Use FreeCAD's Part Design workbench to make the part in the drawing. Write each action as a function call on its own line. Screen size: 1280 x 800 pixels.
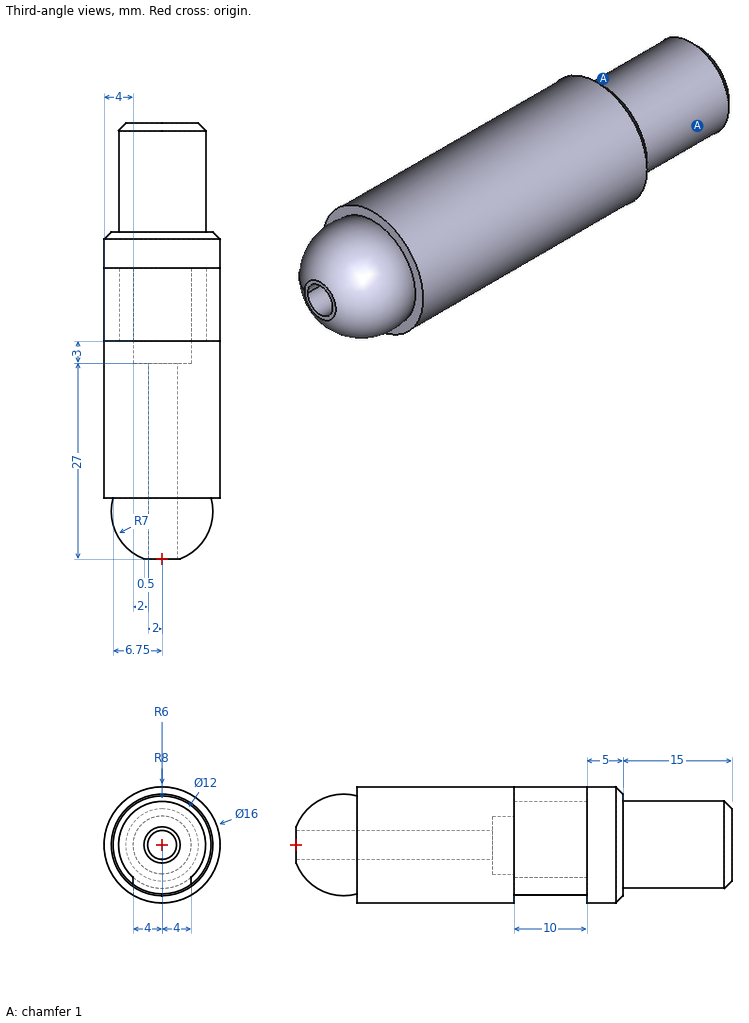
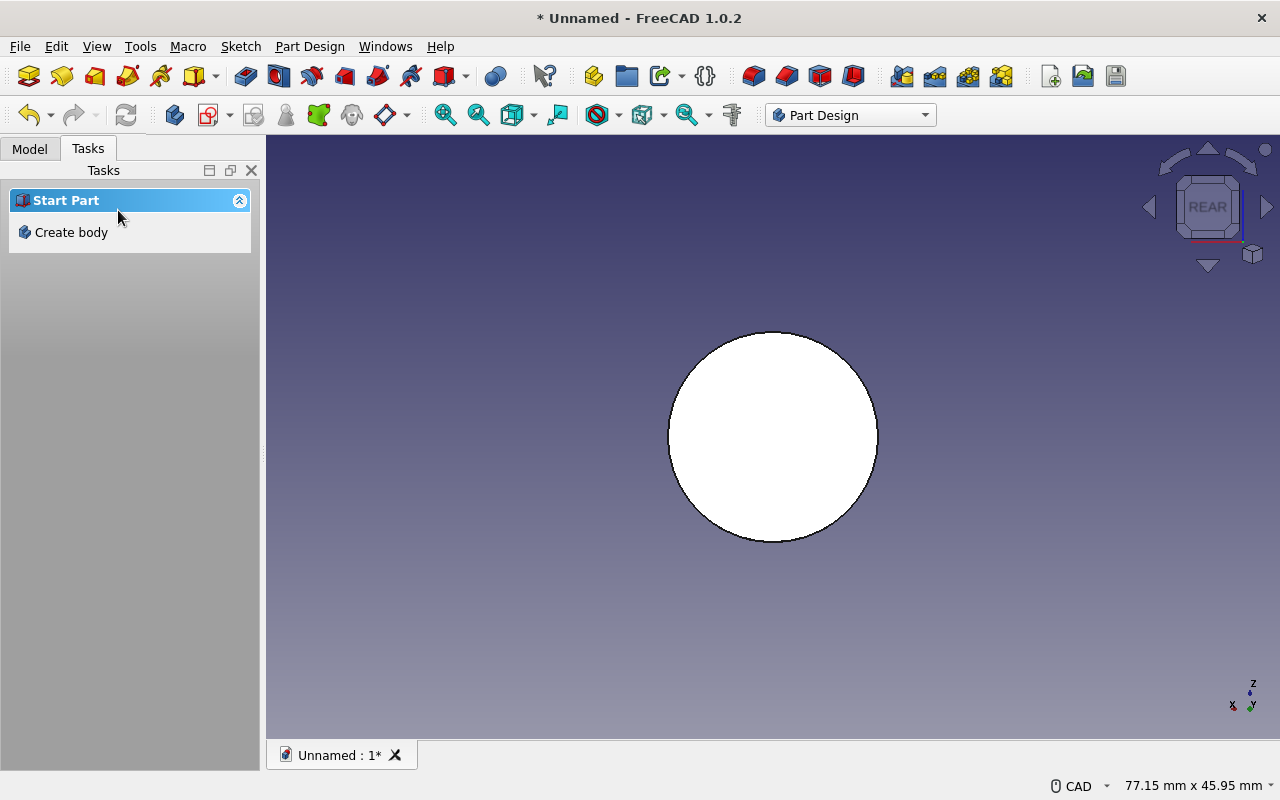
click(446, 116)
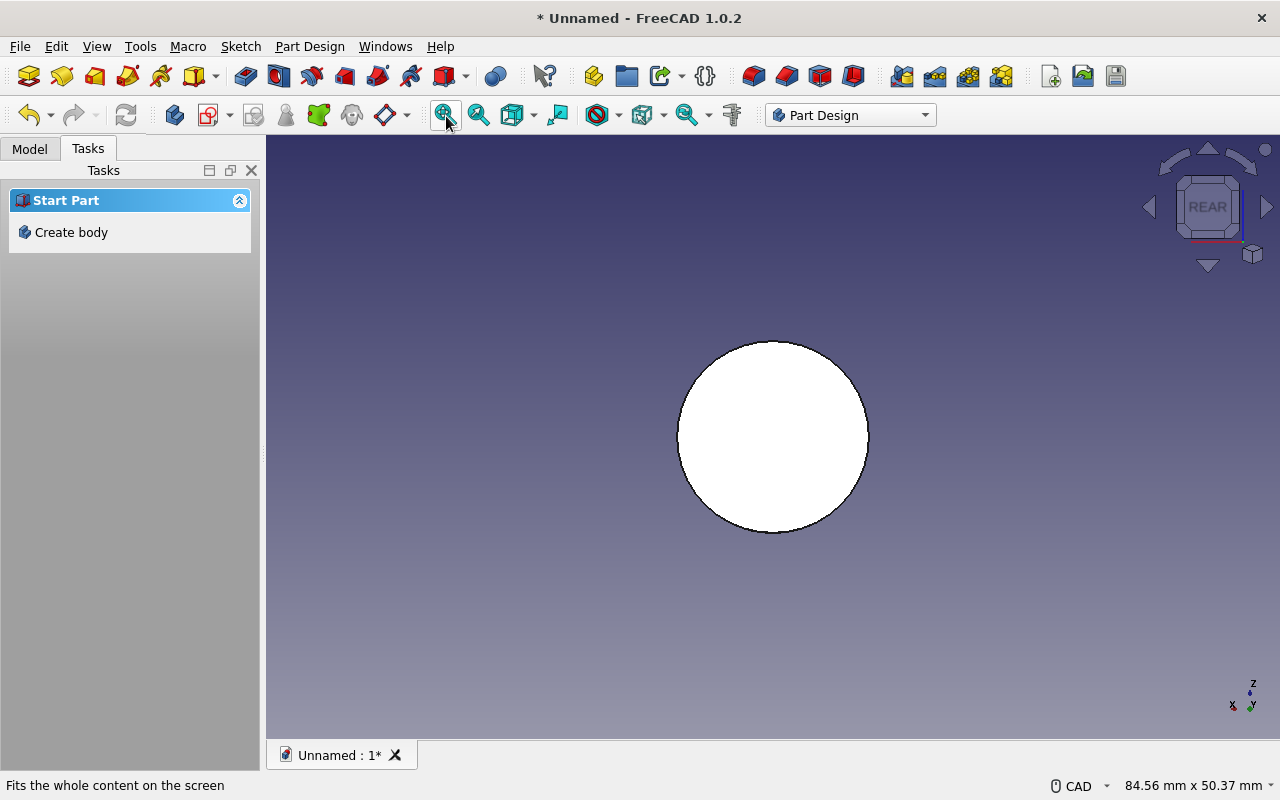
click(773, 436)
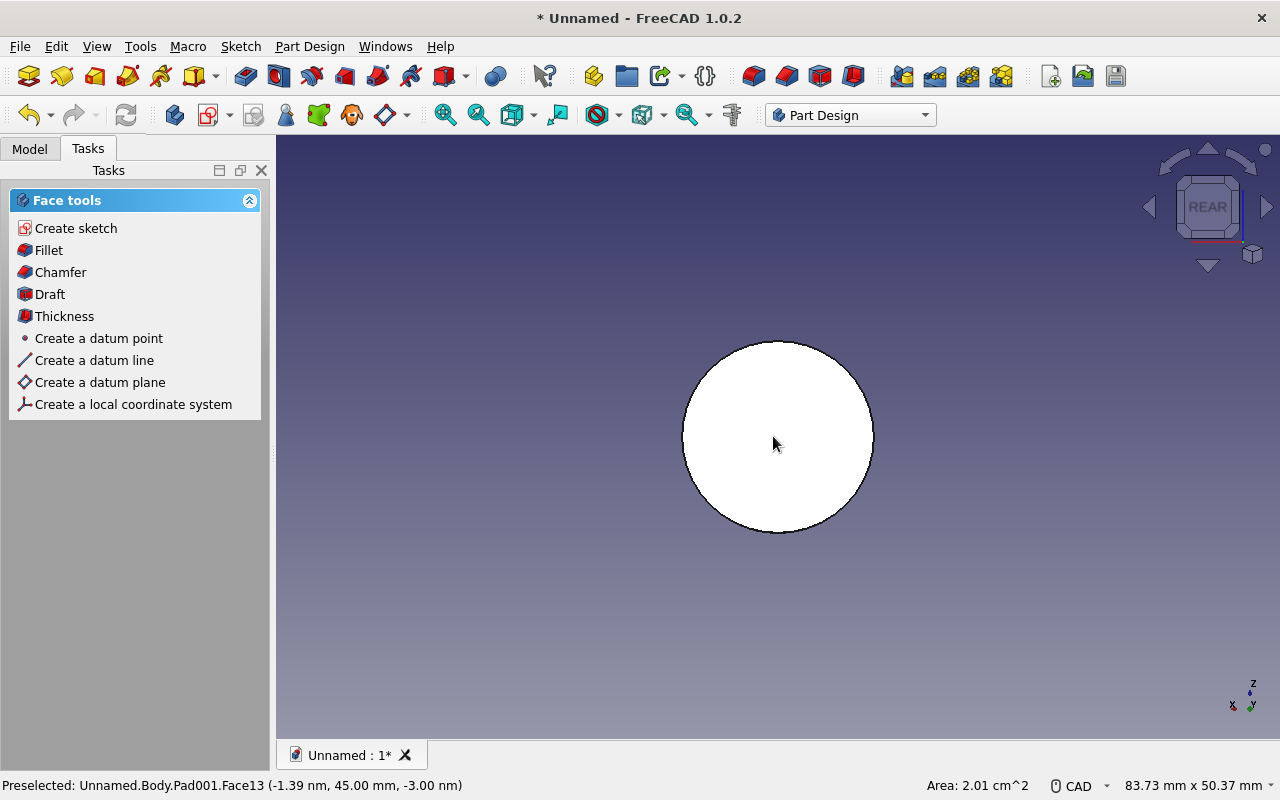
click(208, 116)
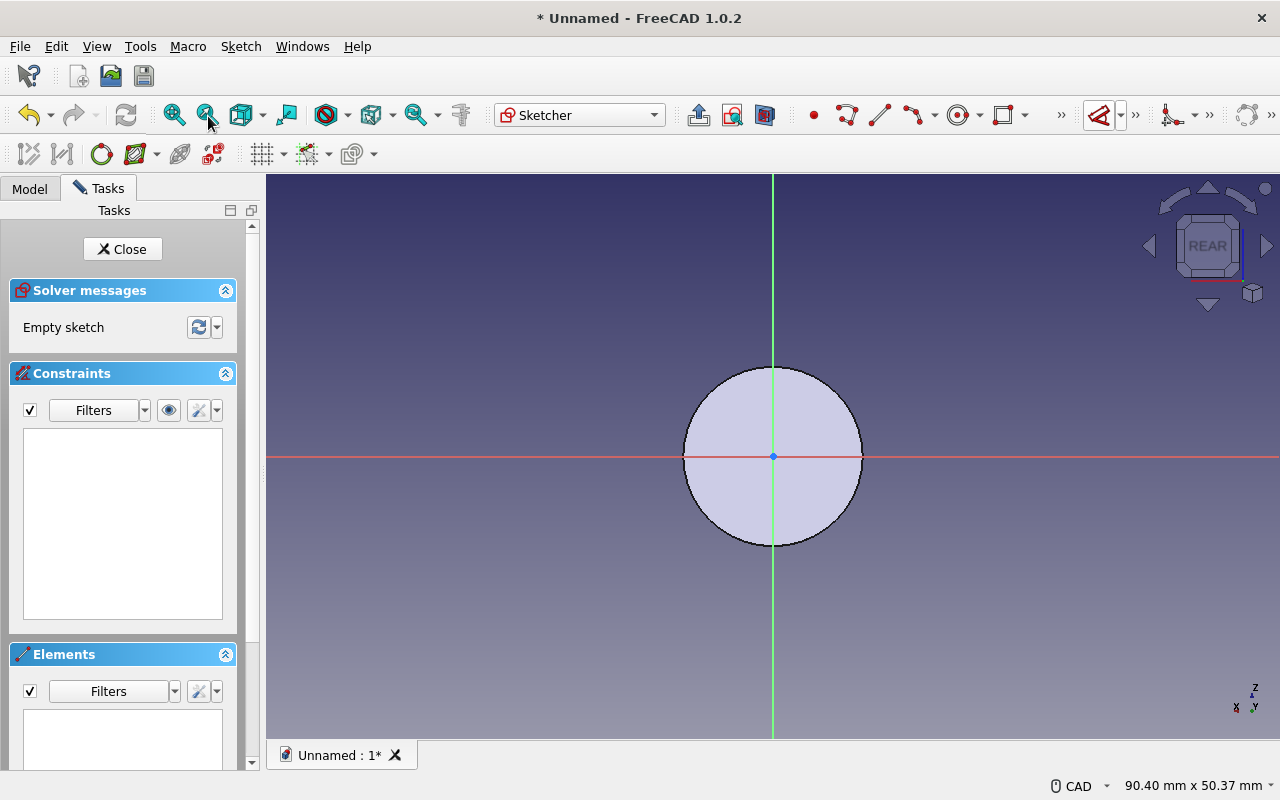
scroll(813, 456, up, 5)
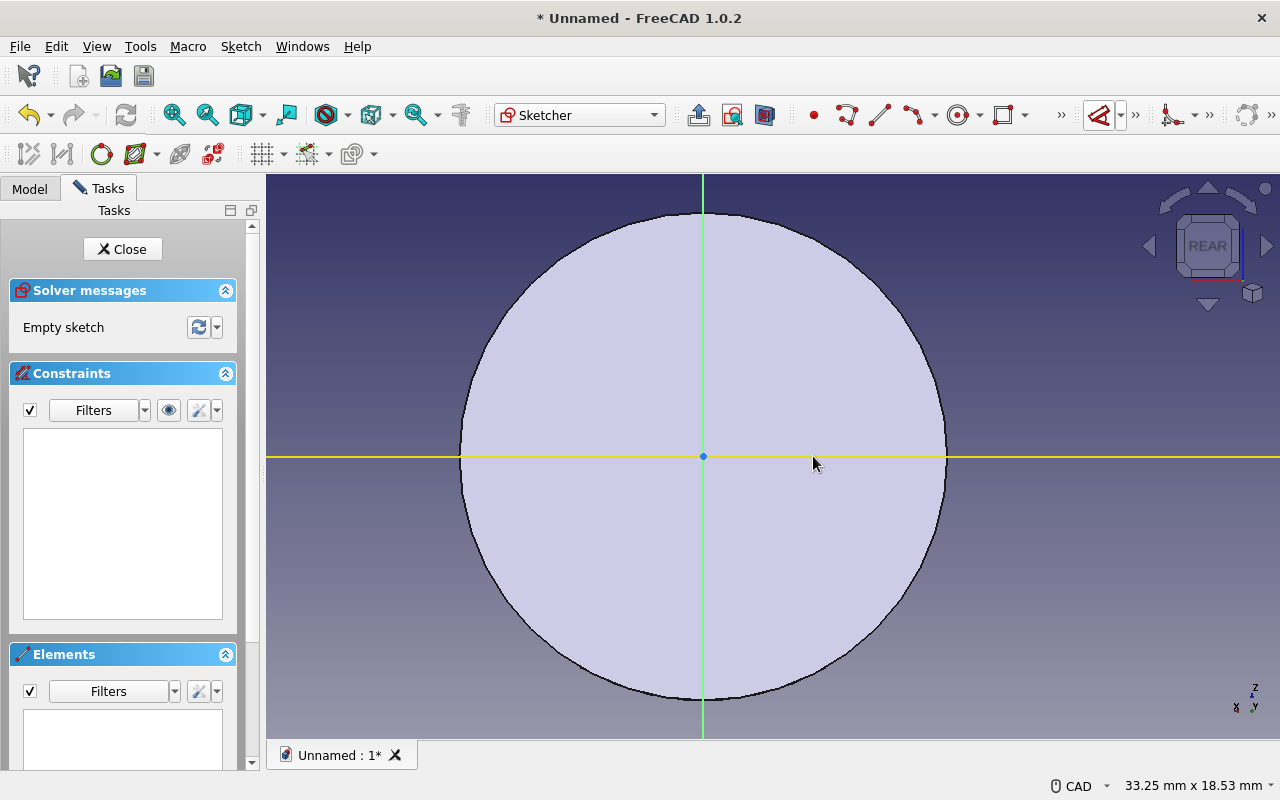
click(958, 116)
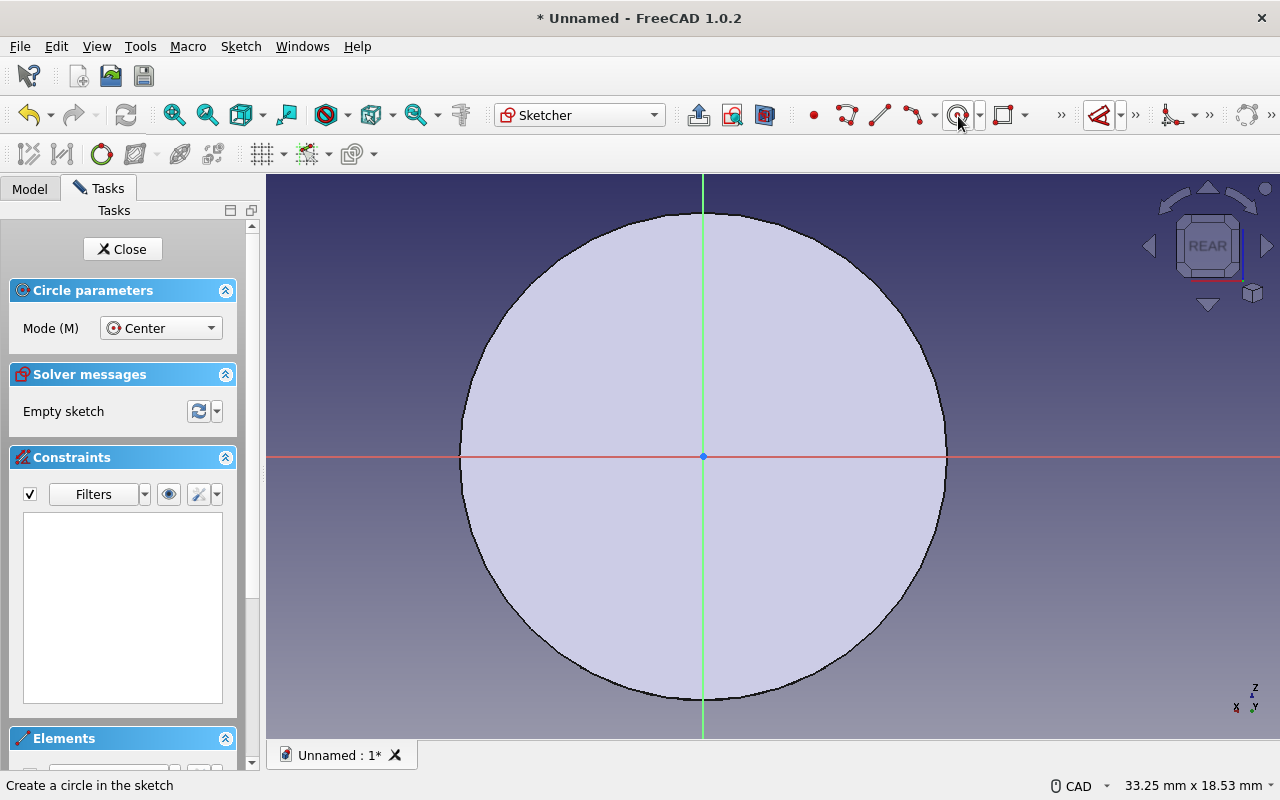
click(703, 456)
click(833, 327)
key(Escape)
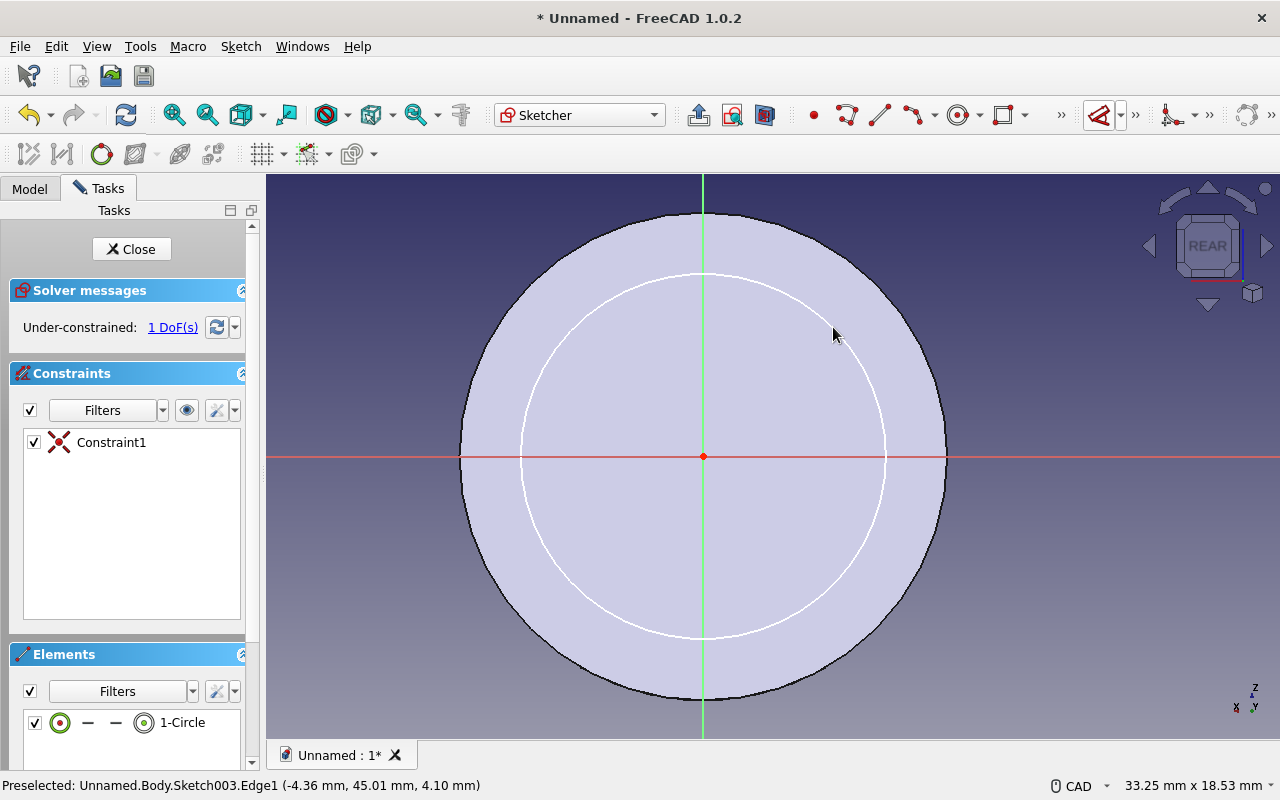
click(832, 327)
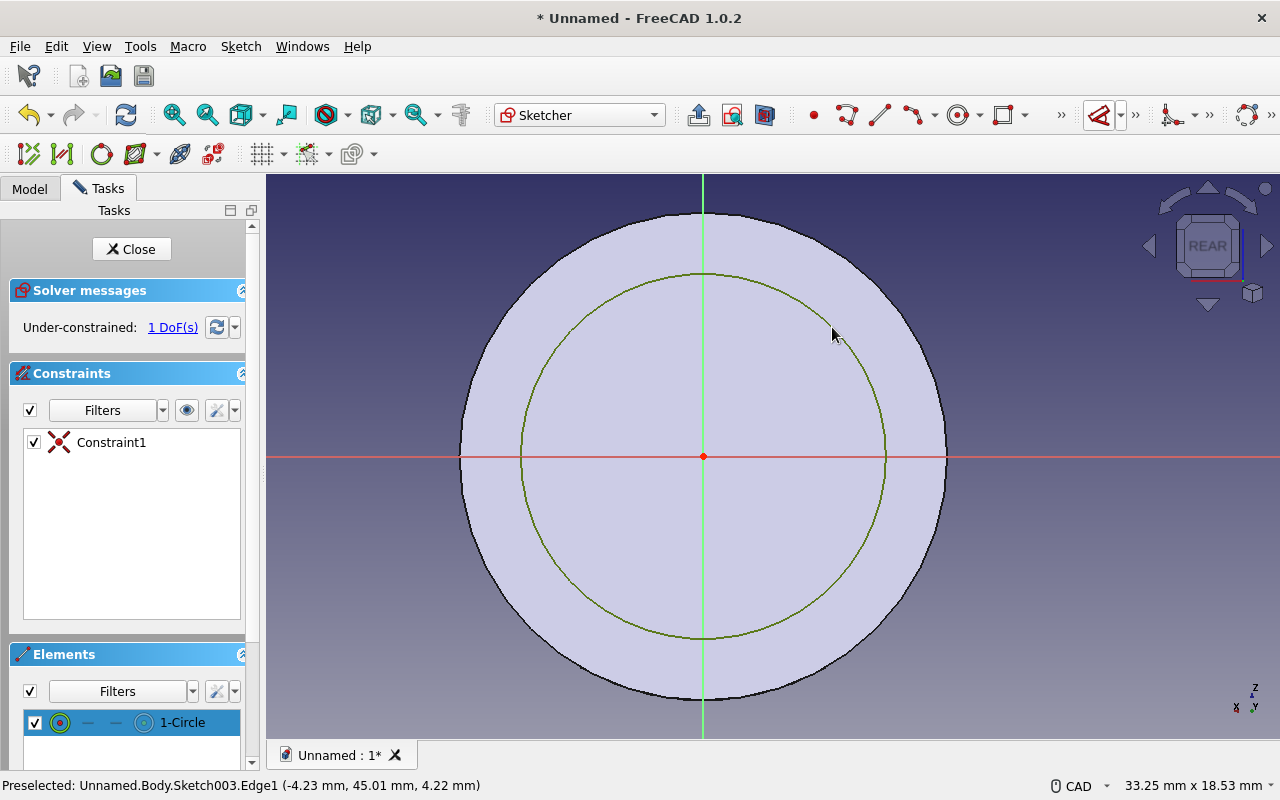
click(1120, 116)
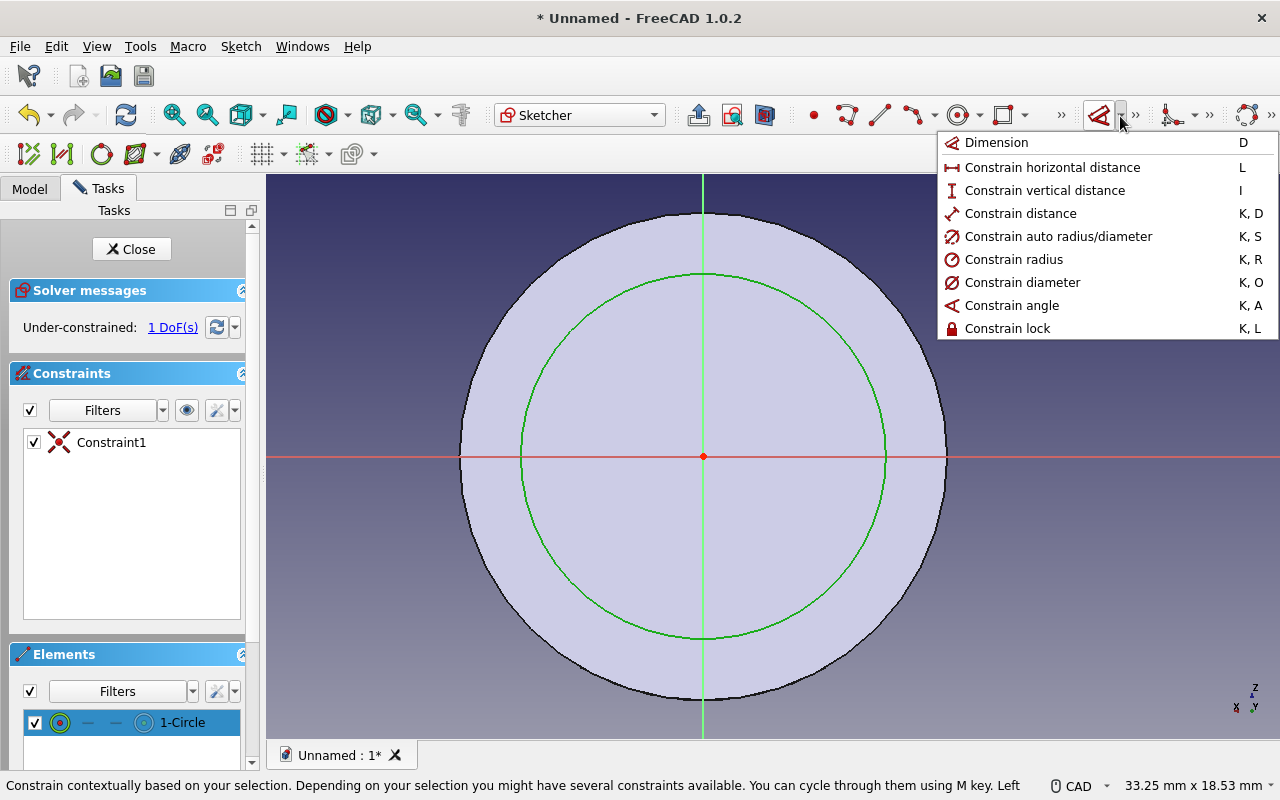
click(1108, 282)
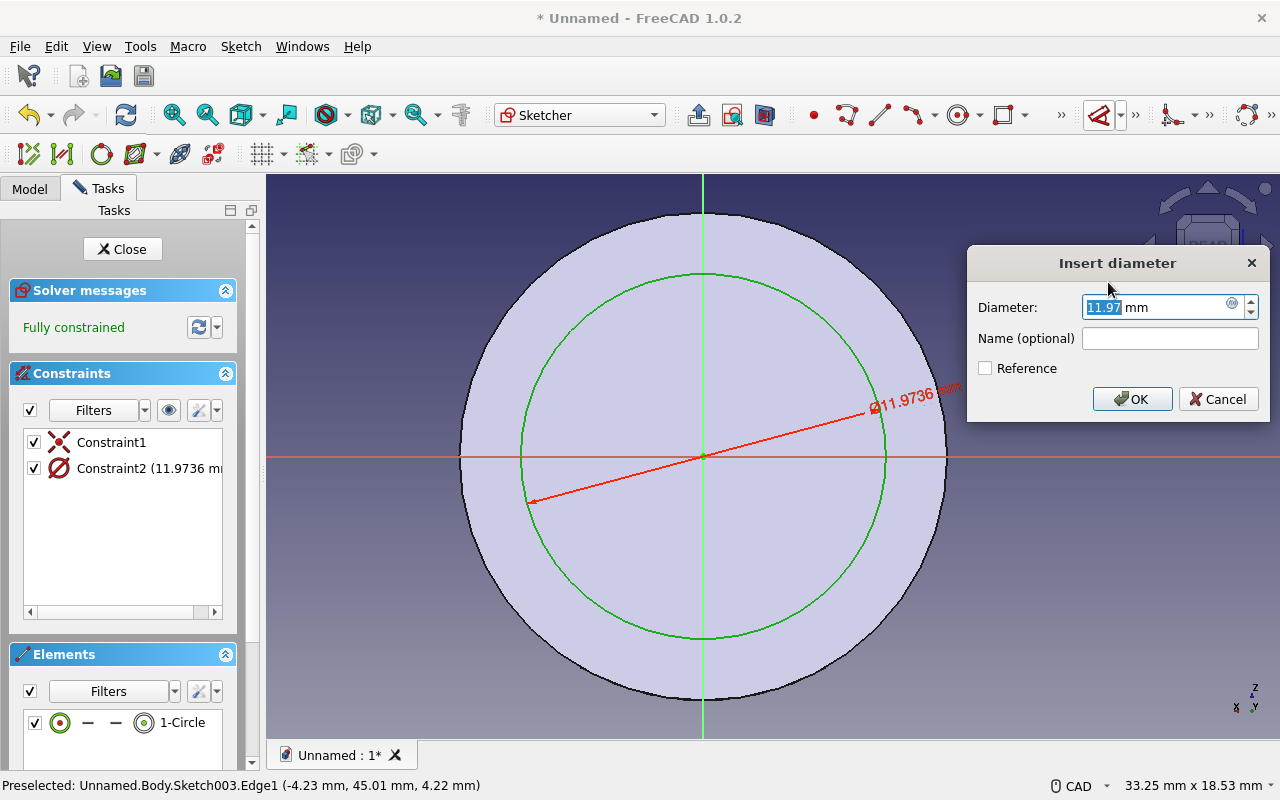
text(12)
key(Return)